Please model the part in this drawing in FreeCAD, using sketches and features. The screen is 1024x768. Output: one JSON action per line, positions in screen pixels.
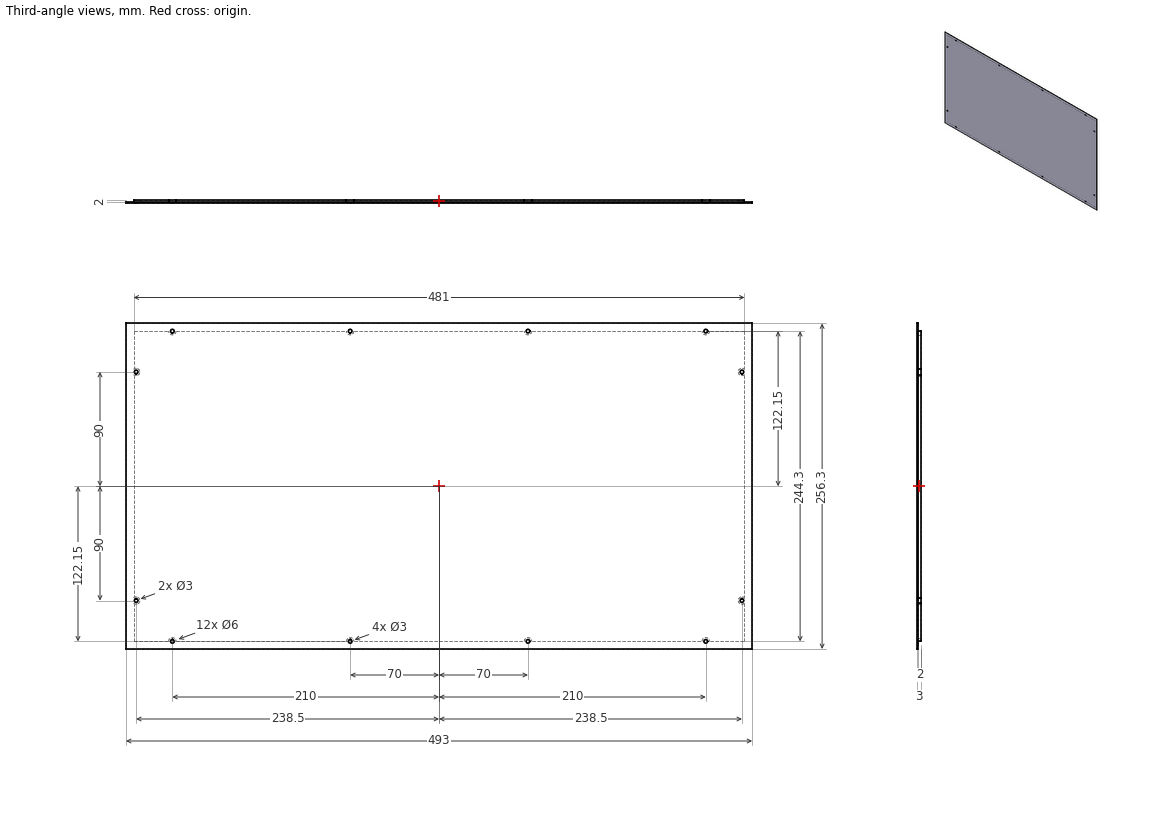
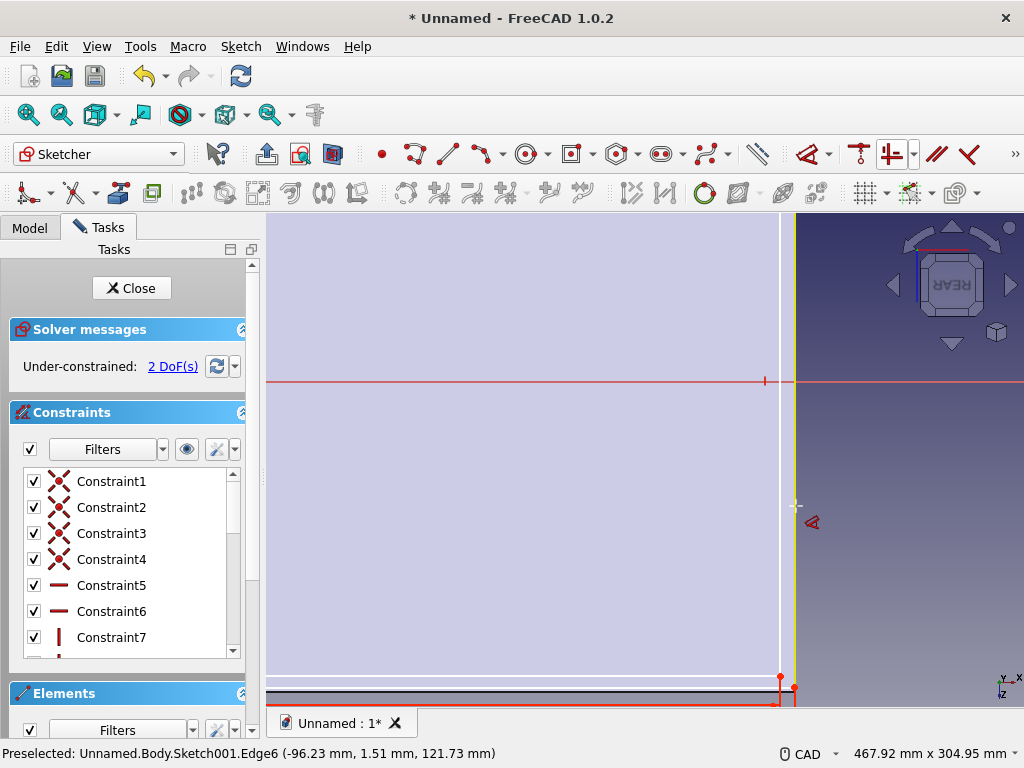
{"action": "left_click", "coordinate": [795, 505]}
{"action": "left_click", "coordinate": [829, 460]}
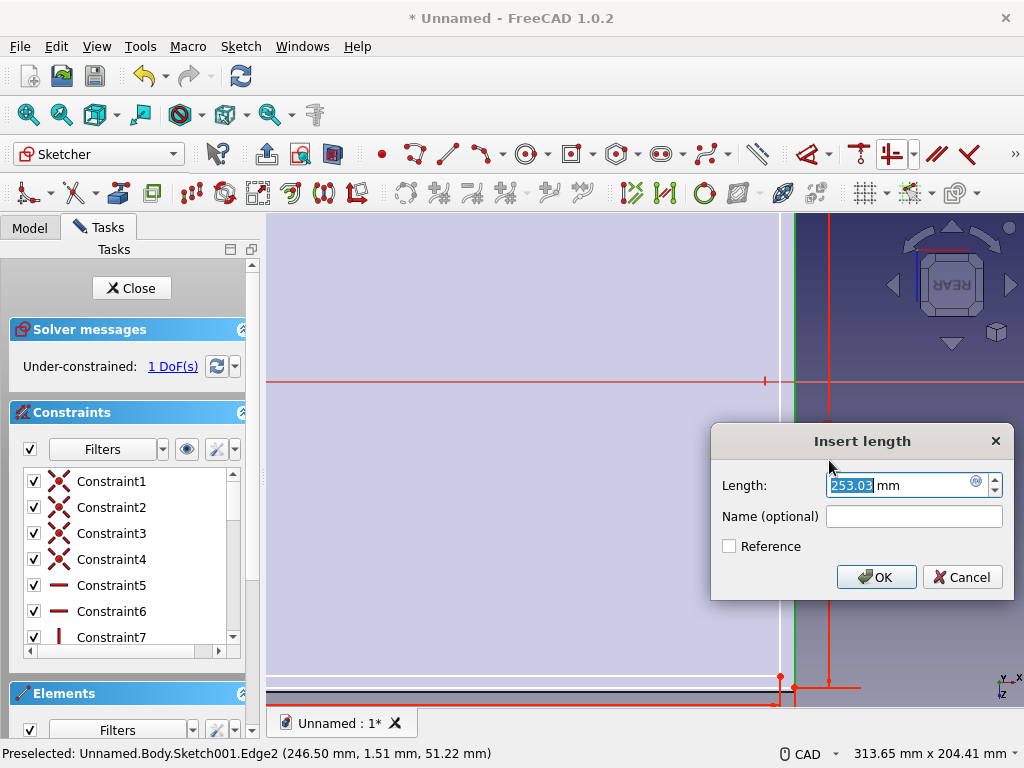
{"action": "type", "text": "256.3"}
{"action": "key", "text": "Return"}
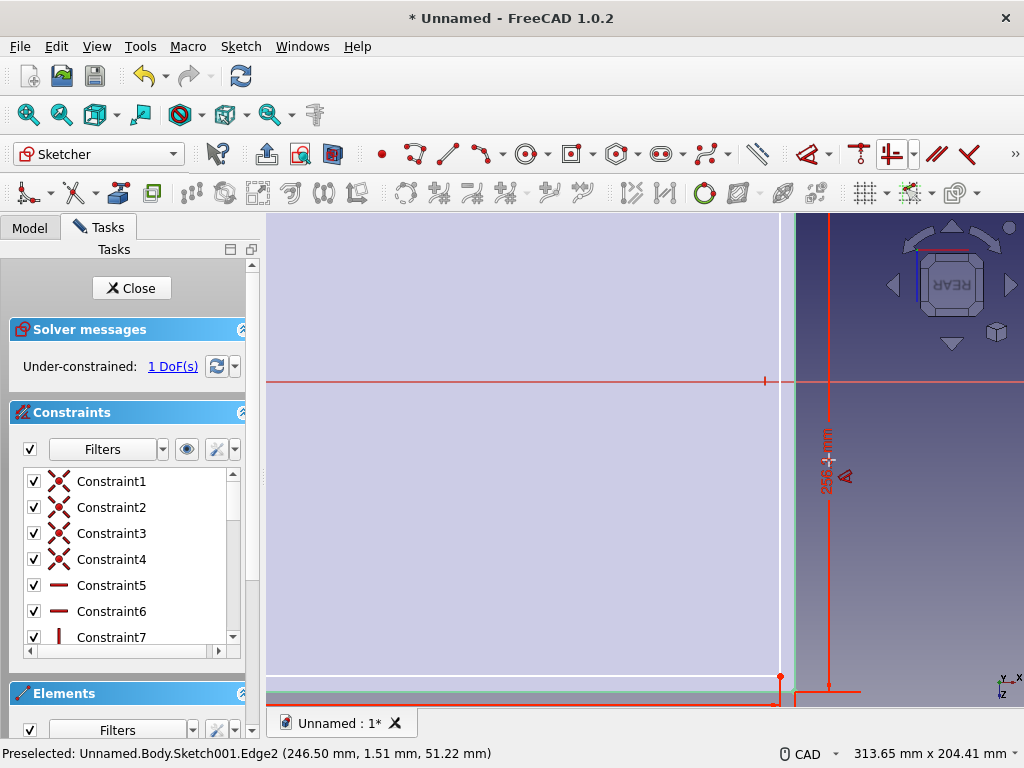
{"action": "left_click", "coordinate": [780, 500]}
{"action": "left_click", "coordinate": [814, 359]}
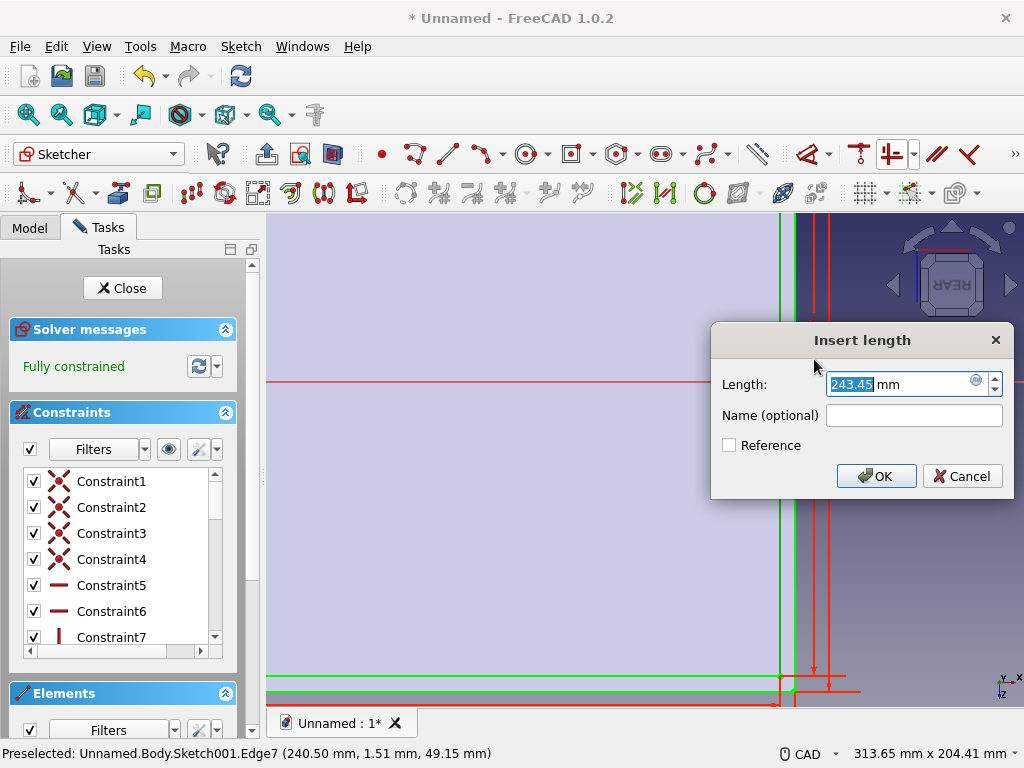
{"action": "type", "text": "244.3"}
{"action": "key", "text": "Return"}
{"action": "key", "text": "Escape"}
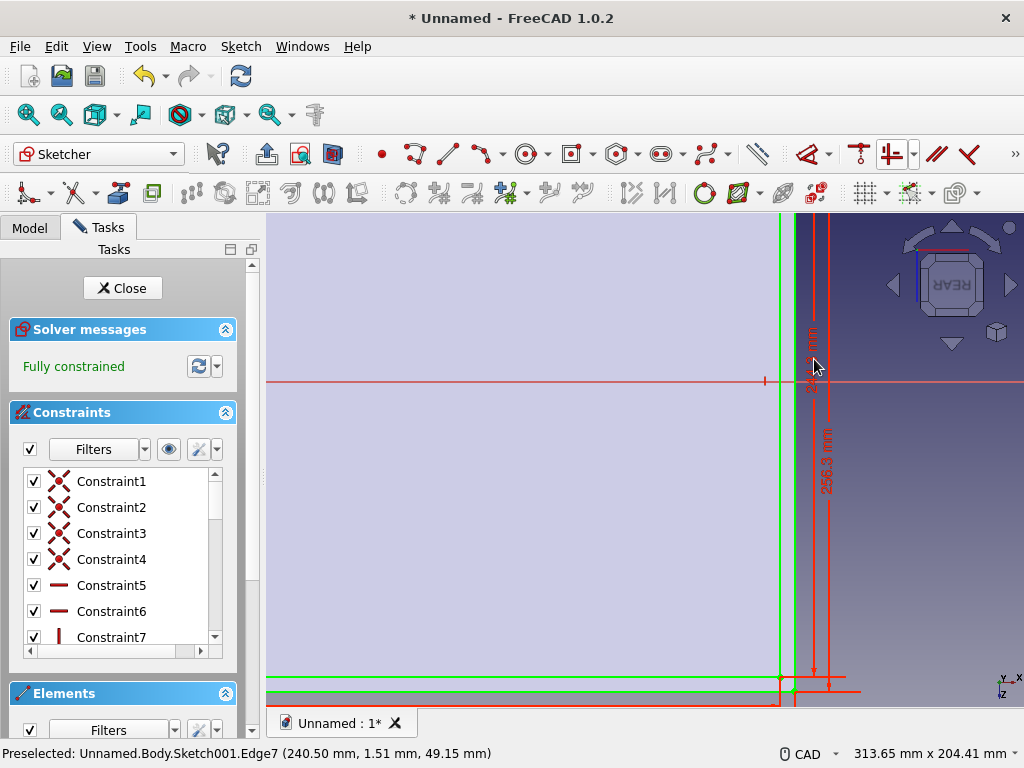
{"action": "left_click", "coordinate": [123, 288]}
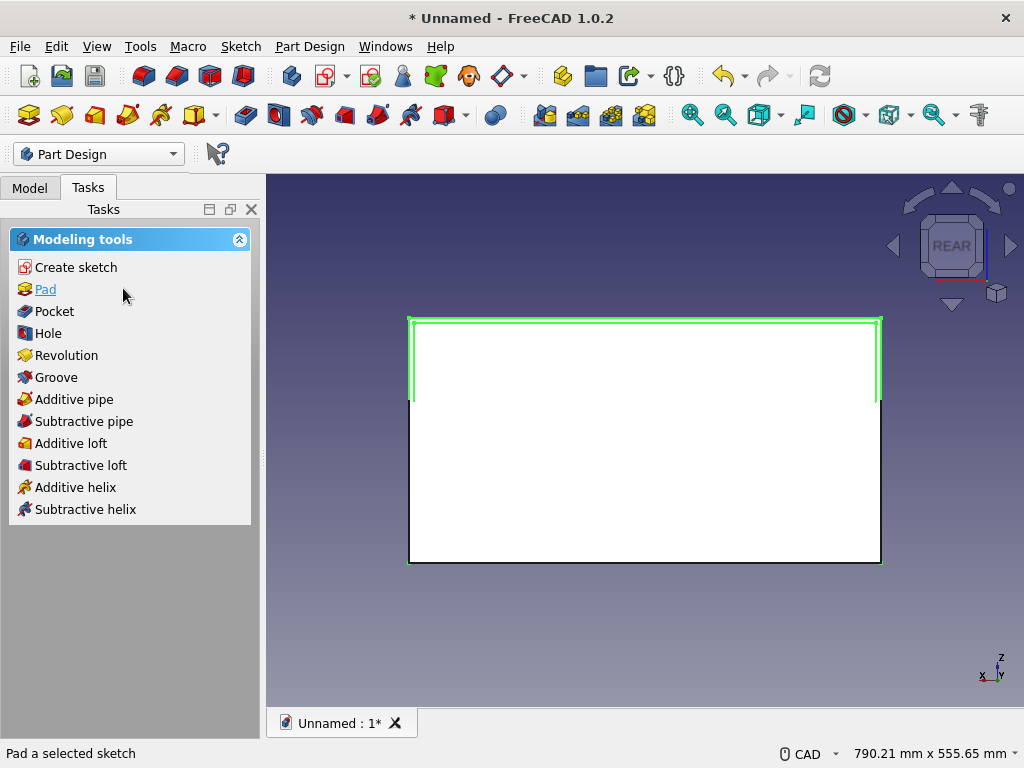
{"action": "left_click", "coordinate": [246, 116]}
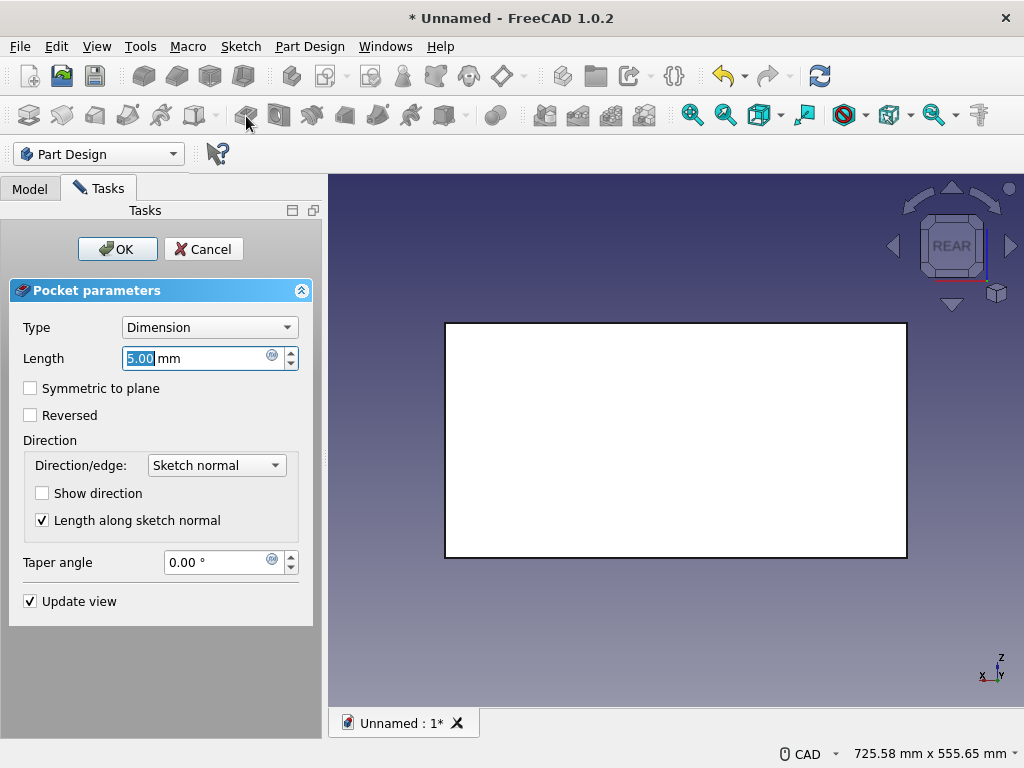
{"action": "type", "text": "2"}
{"action": "key", "text": "Tab"}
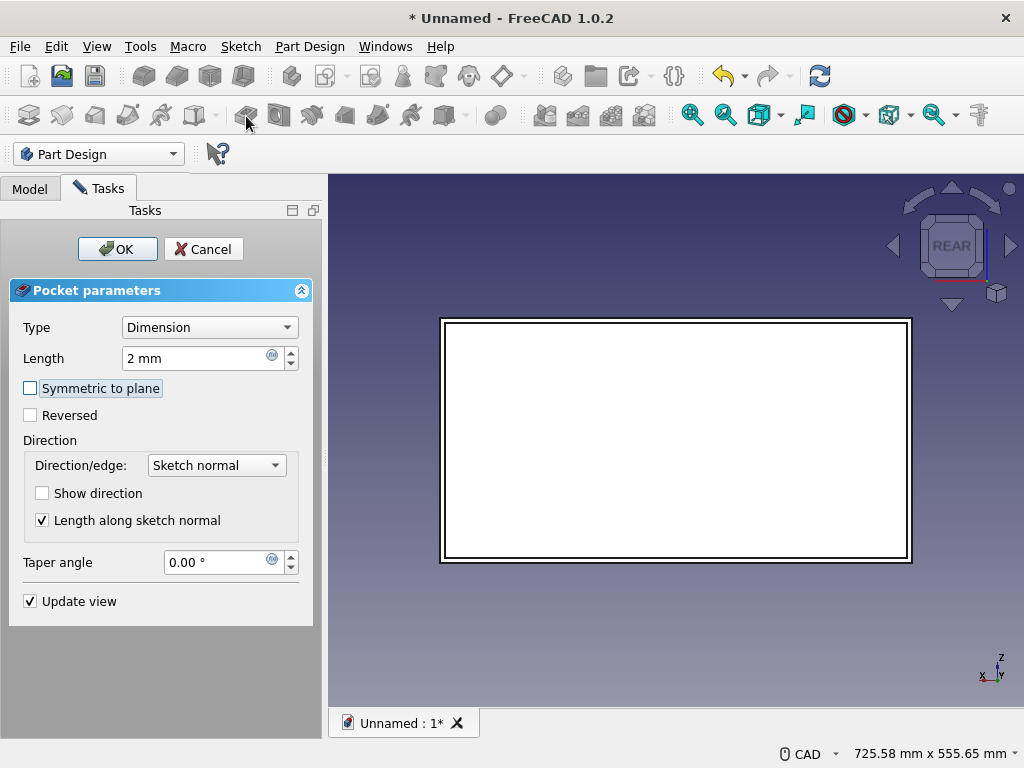
{"action": "left_click", "coordinate": [118, 249]}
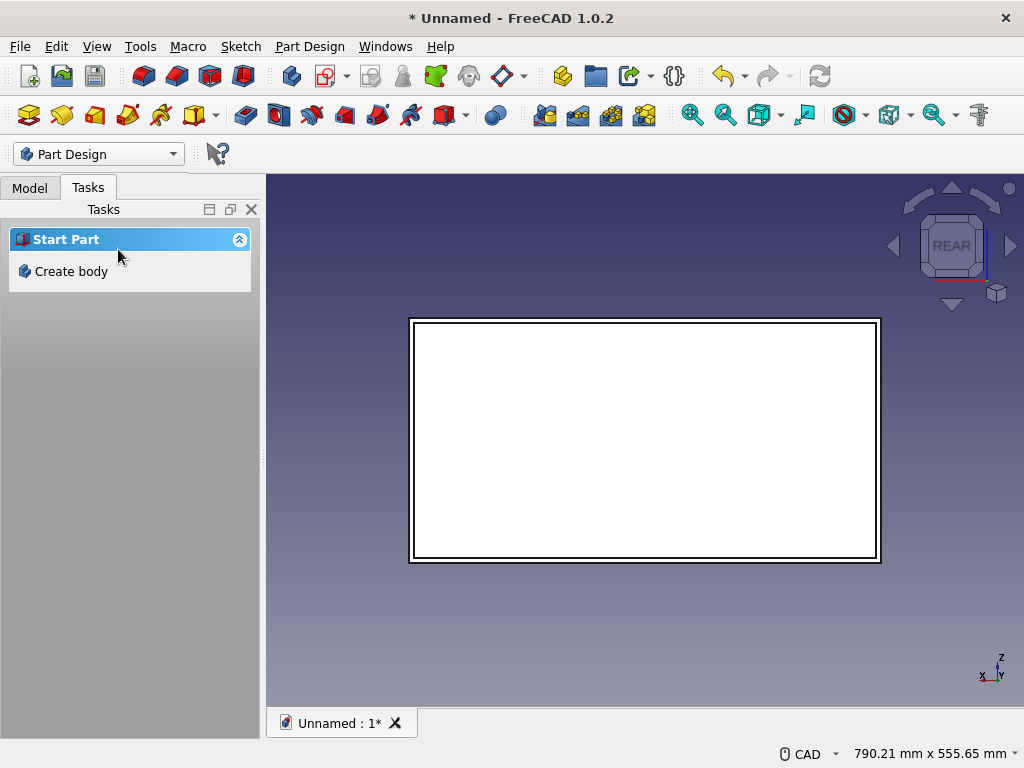
{"action": "left_click", "coordinate": [579, 440]}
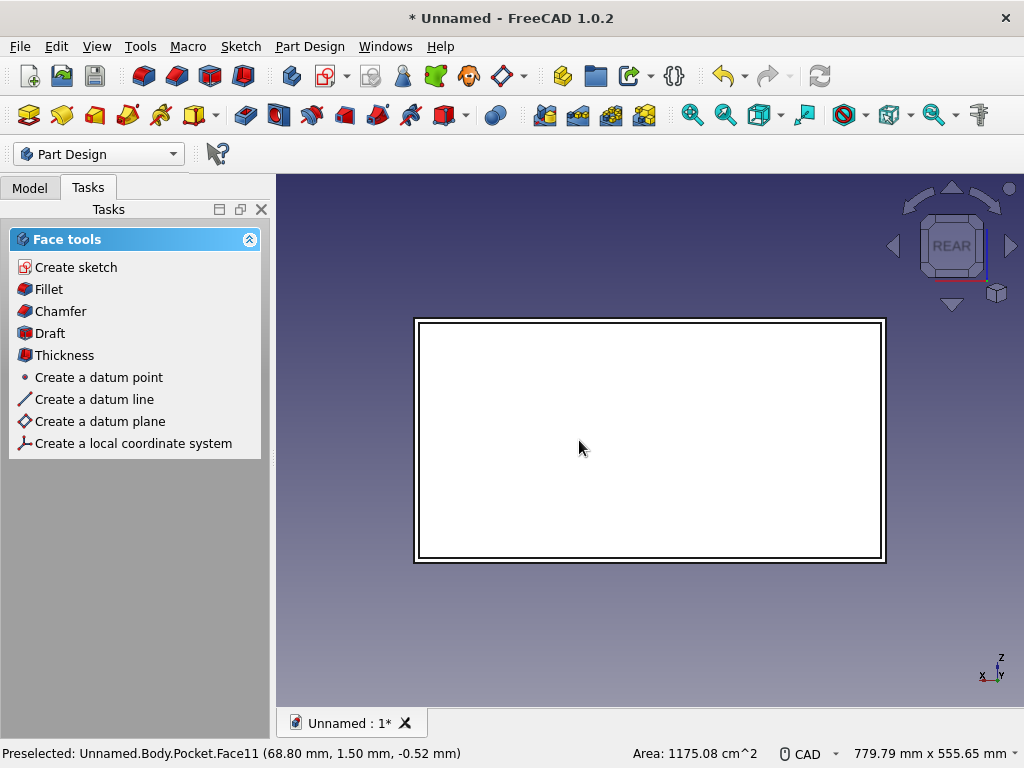
{"action": "left_click", "coordinate": [324, 76]}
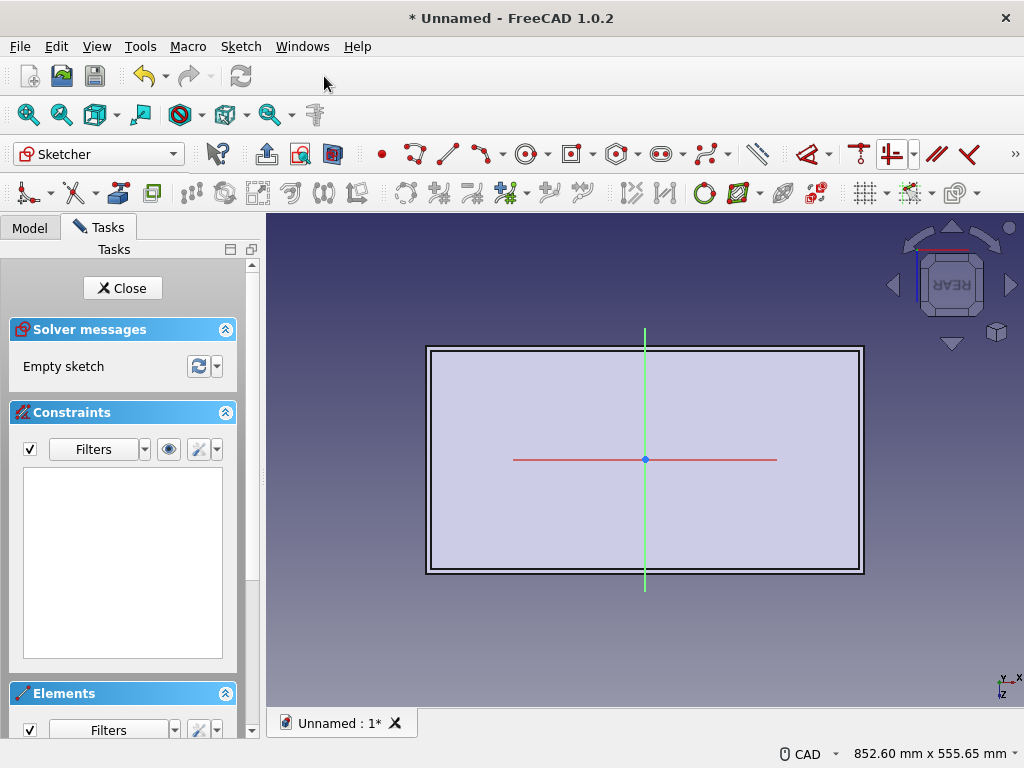
{"action": "left_click", "coordinate": [526, 154]}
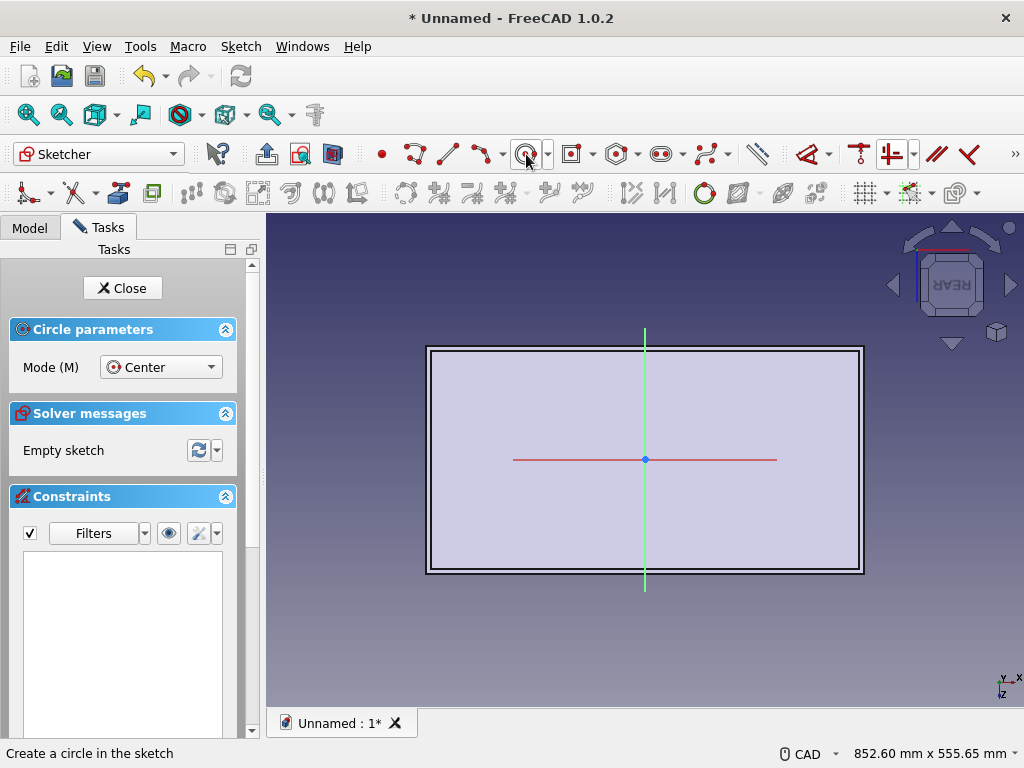
{"action": "scroll", "coordinate": [583, 351], "scroll_direction": "up", "scroll_amount": 15}